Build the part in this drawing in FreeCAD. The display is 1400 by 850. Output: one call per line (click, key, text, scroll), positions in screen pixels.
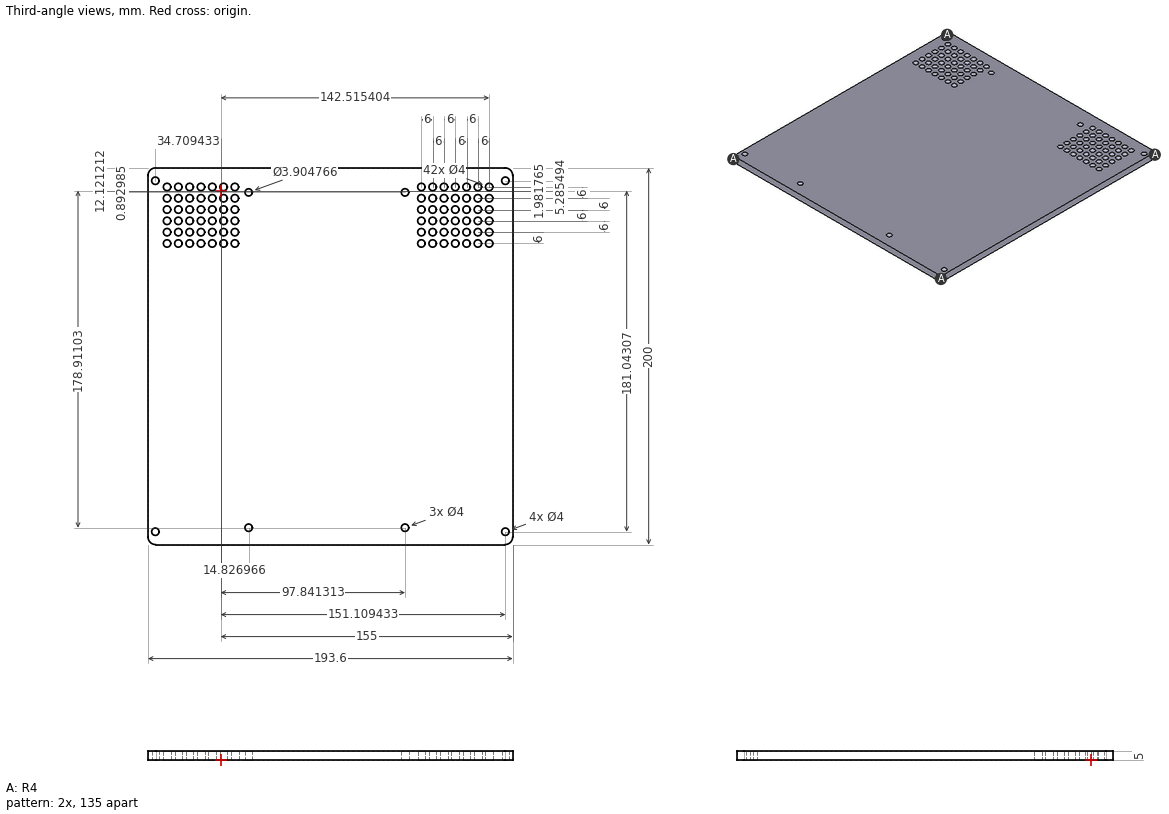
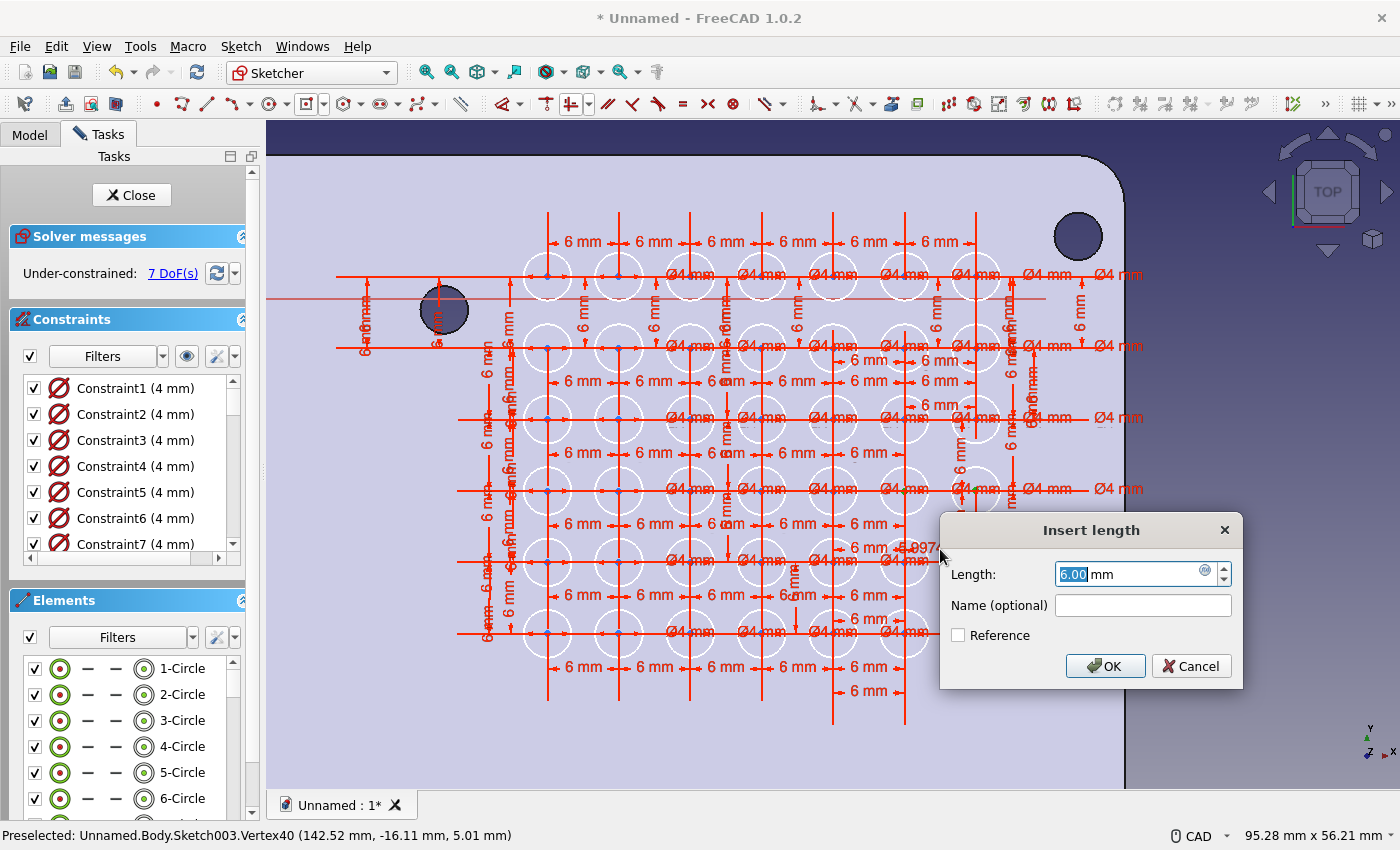
text(6)
key(Return)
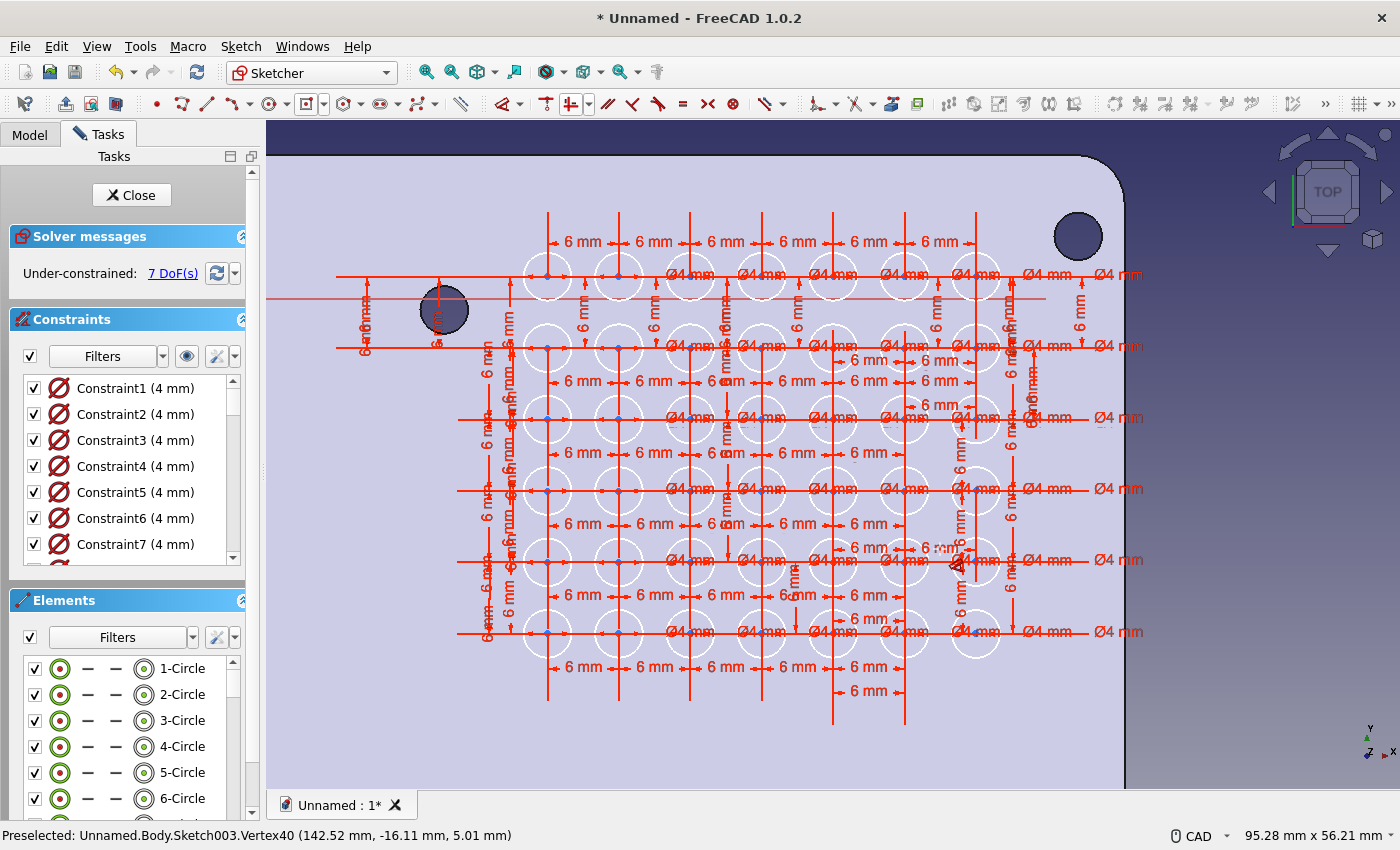
click(976, 420)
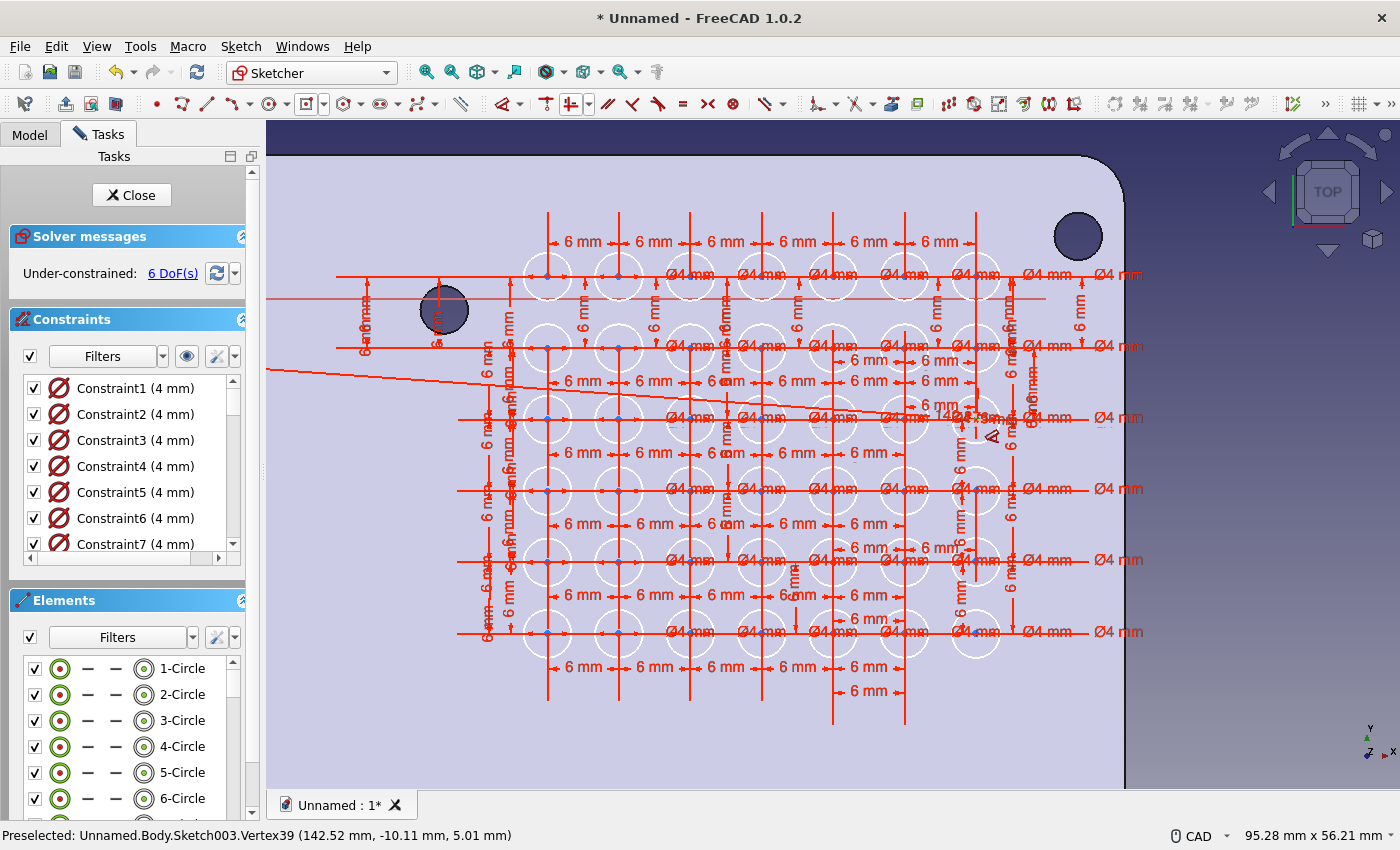
click(976, 491)
click(1034, 455)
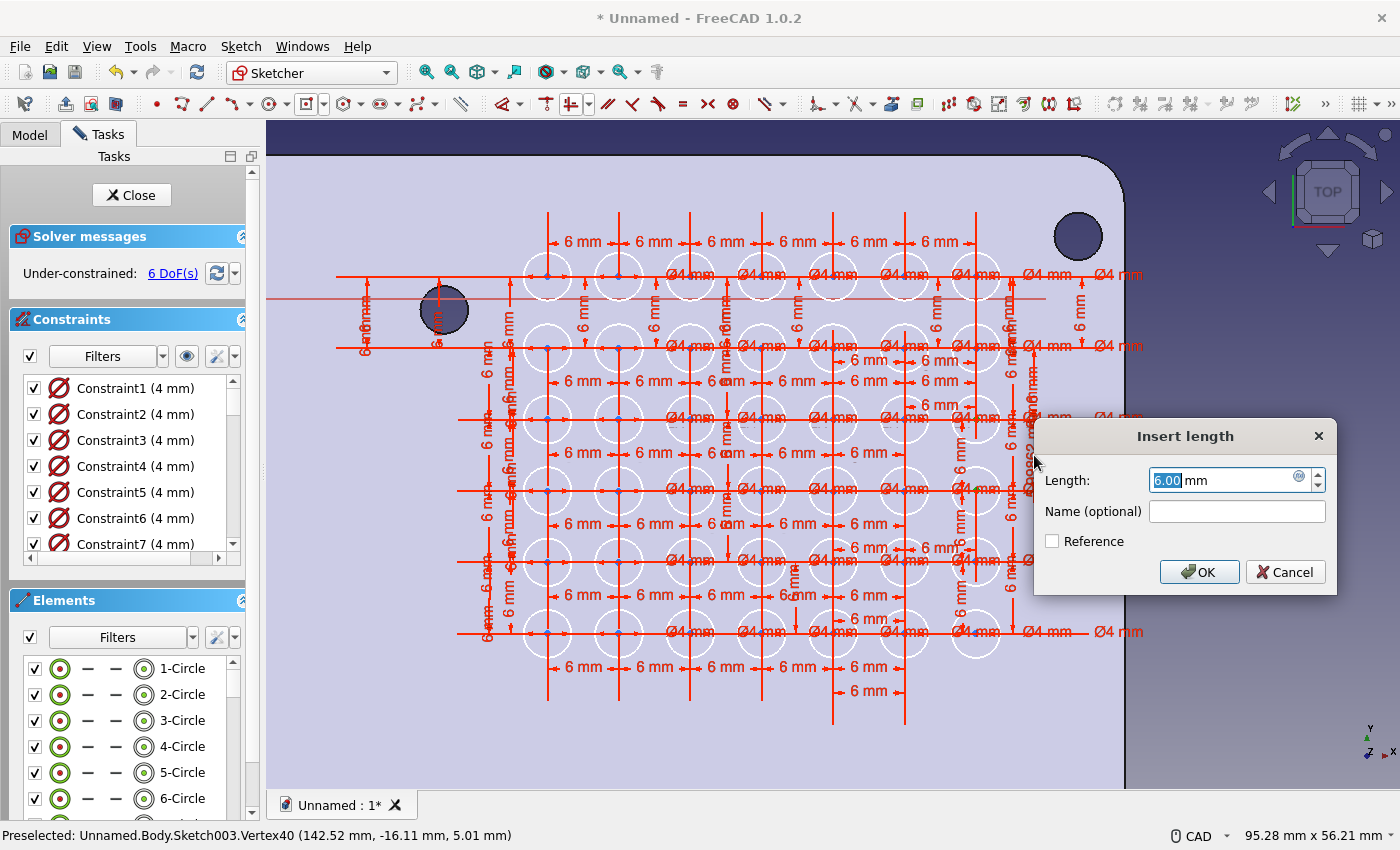
text(6)
key(Return)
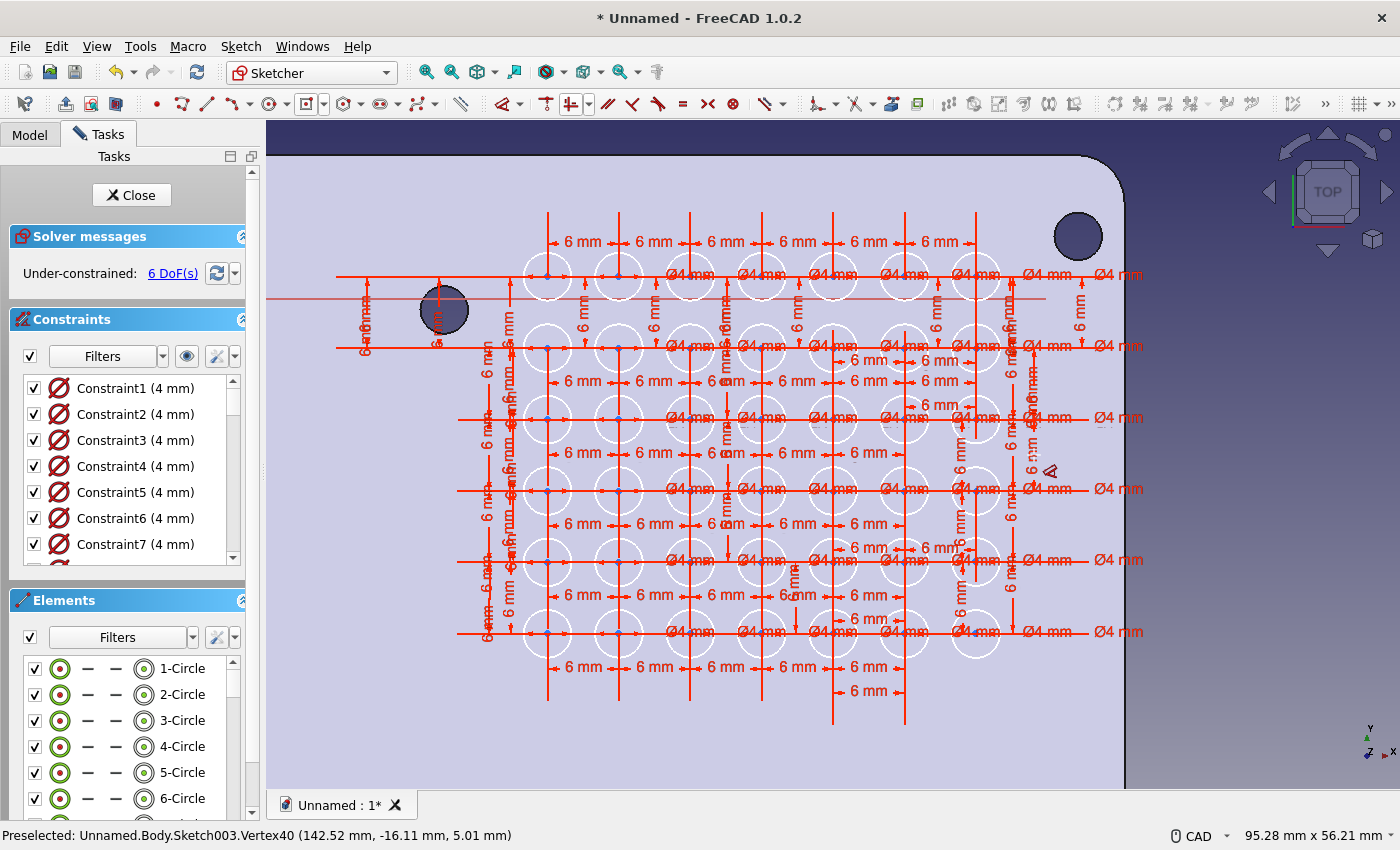
click(905, 562)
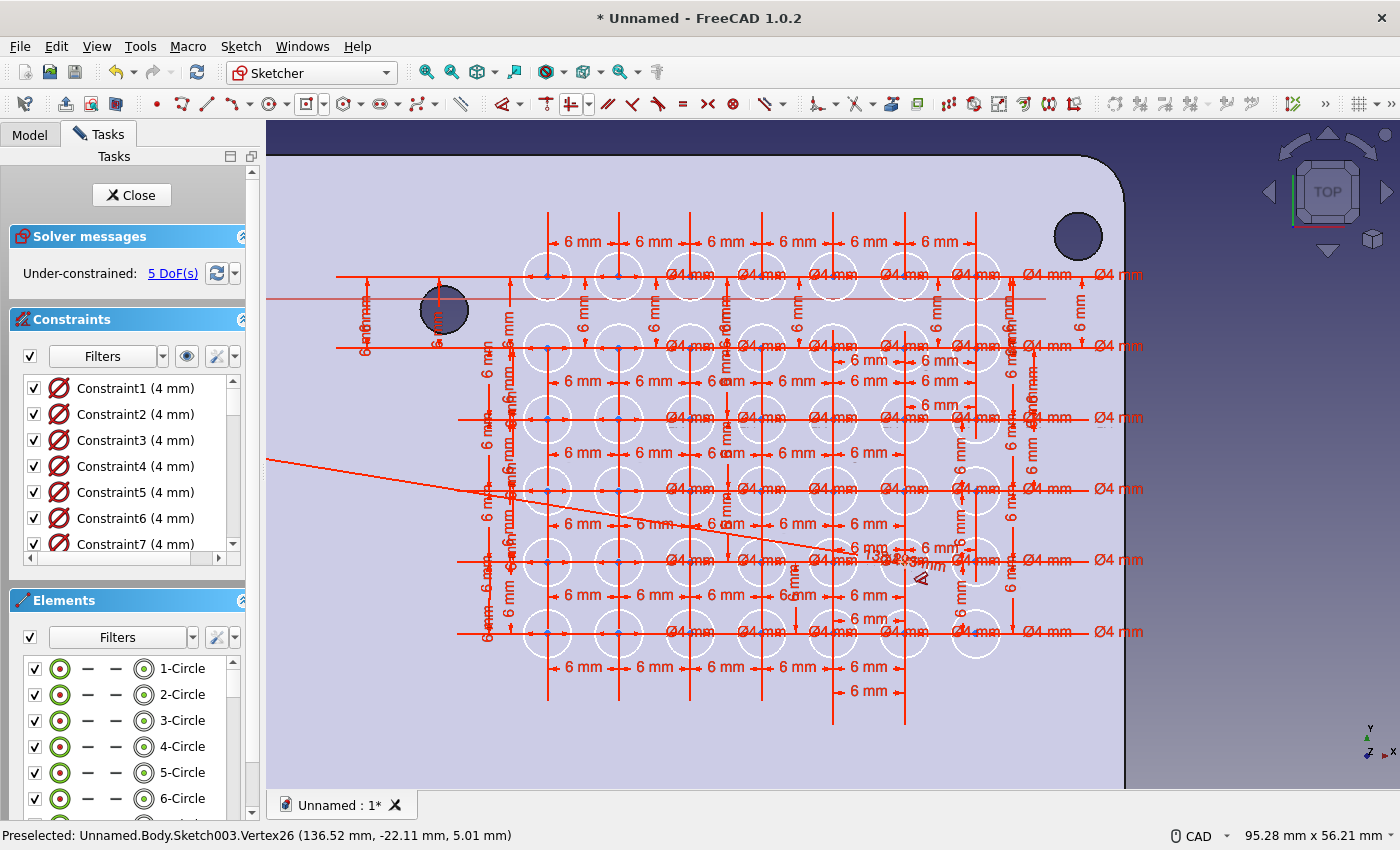
click(976, 562)
click(940, 620)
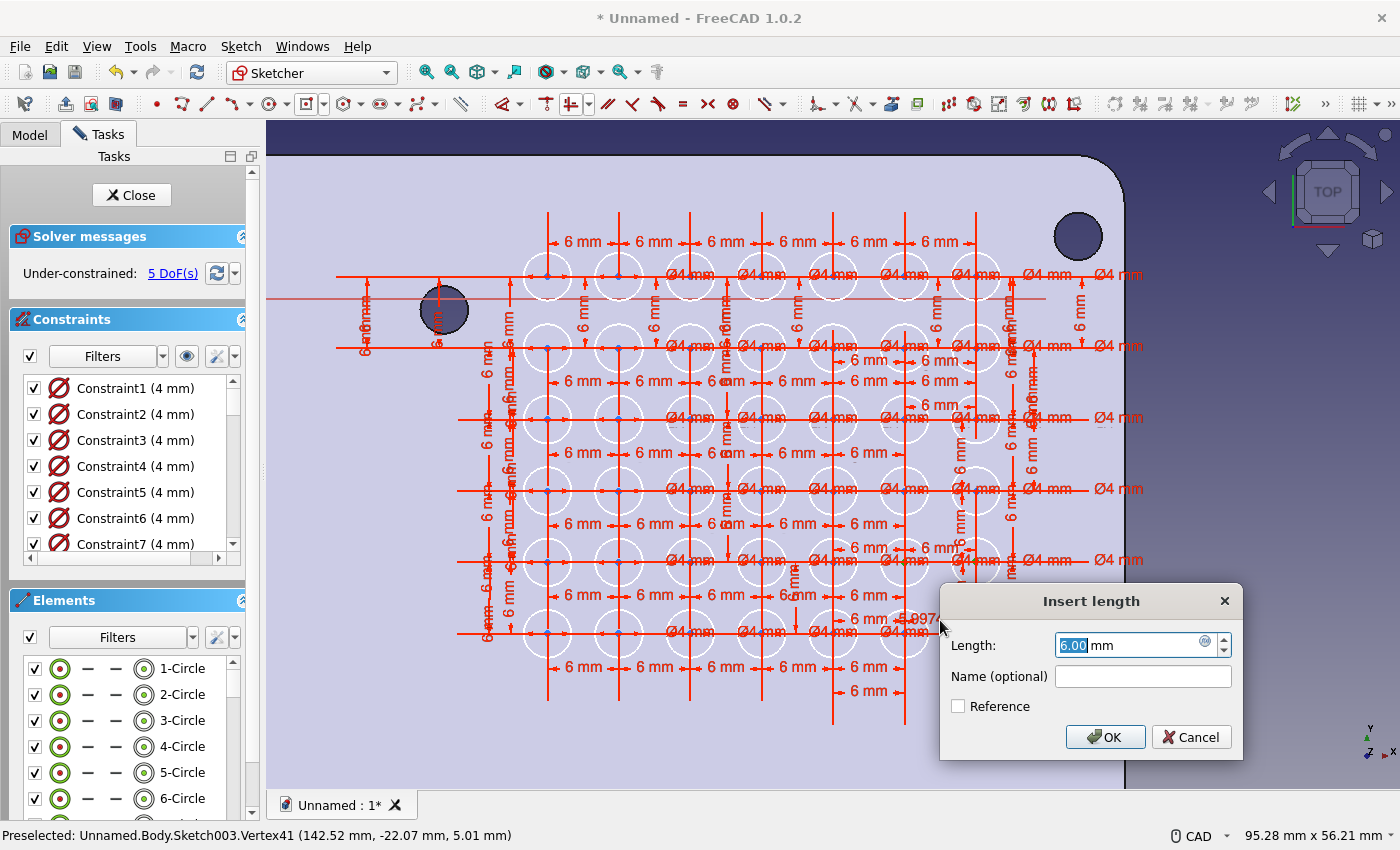
text(6)
key(Return)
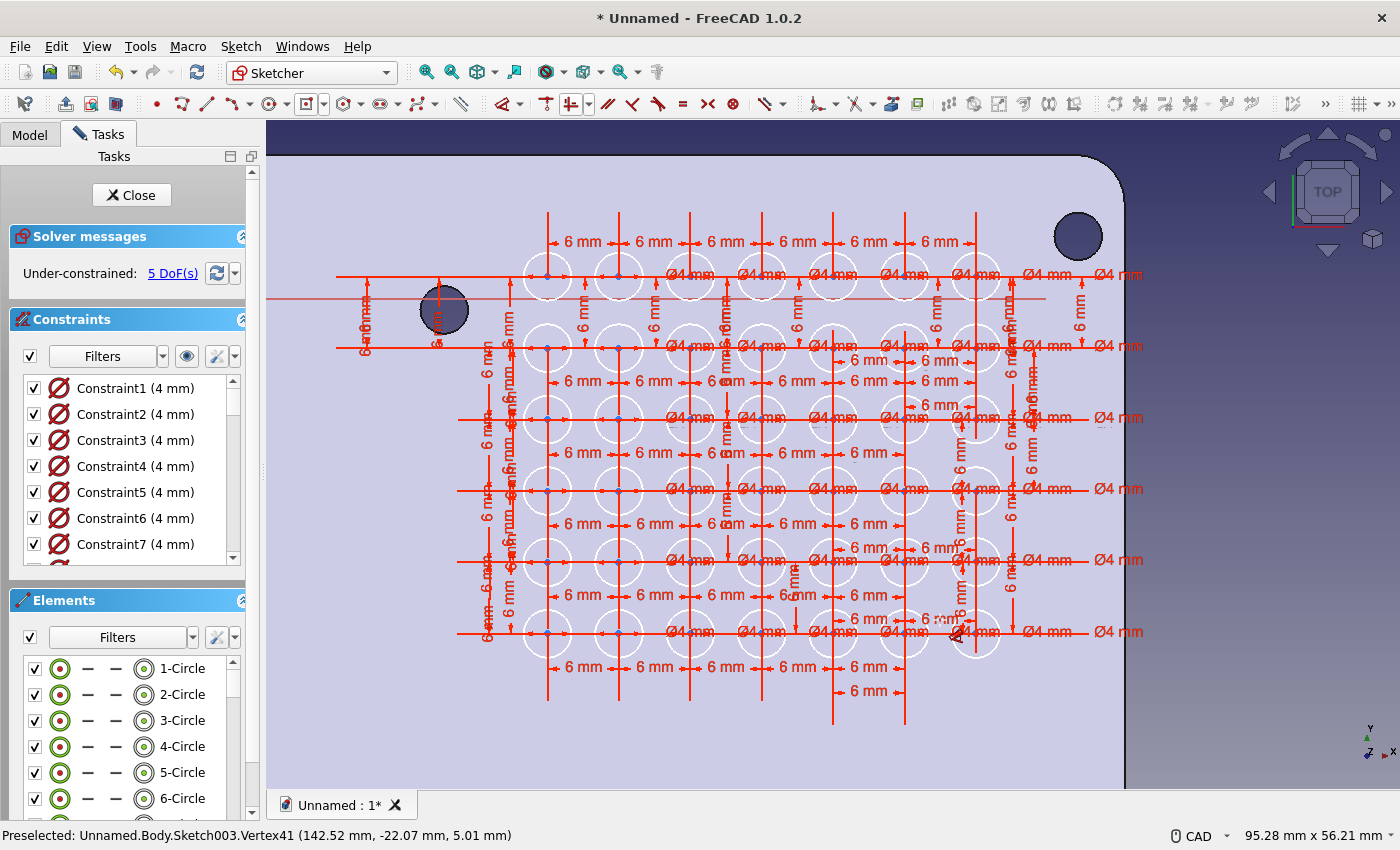
click(976, 491)